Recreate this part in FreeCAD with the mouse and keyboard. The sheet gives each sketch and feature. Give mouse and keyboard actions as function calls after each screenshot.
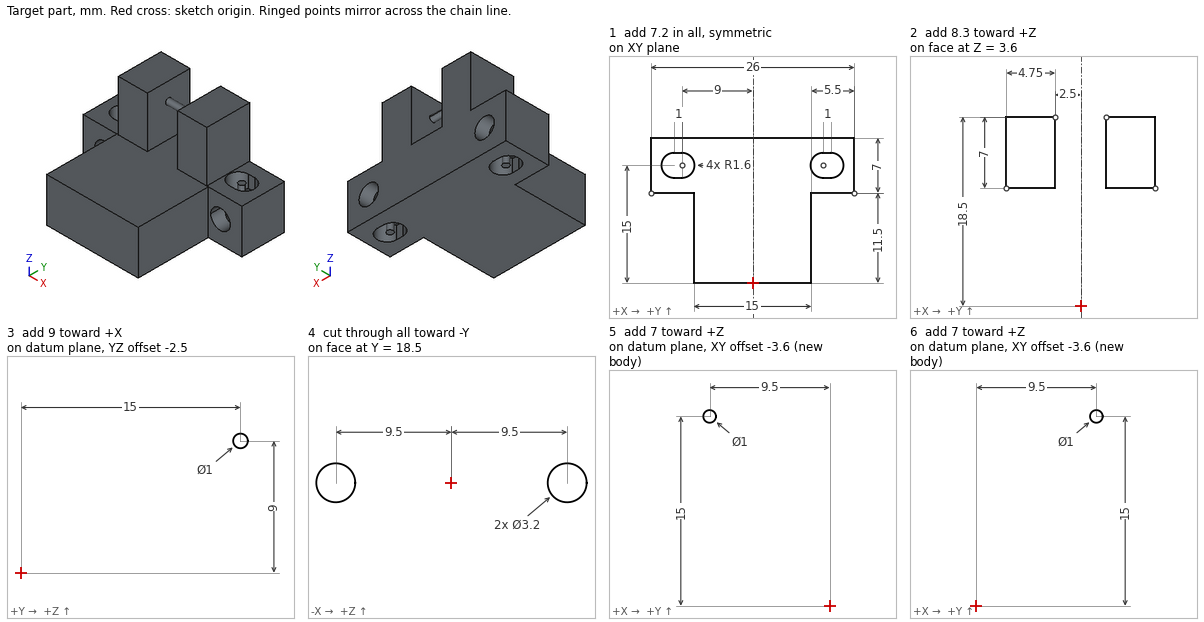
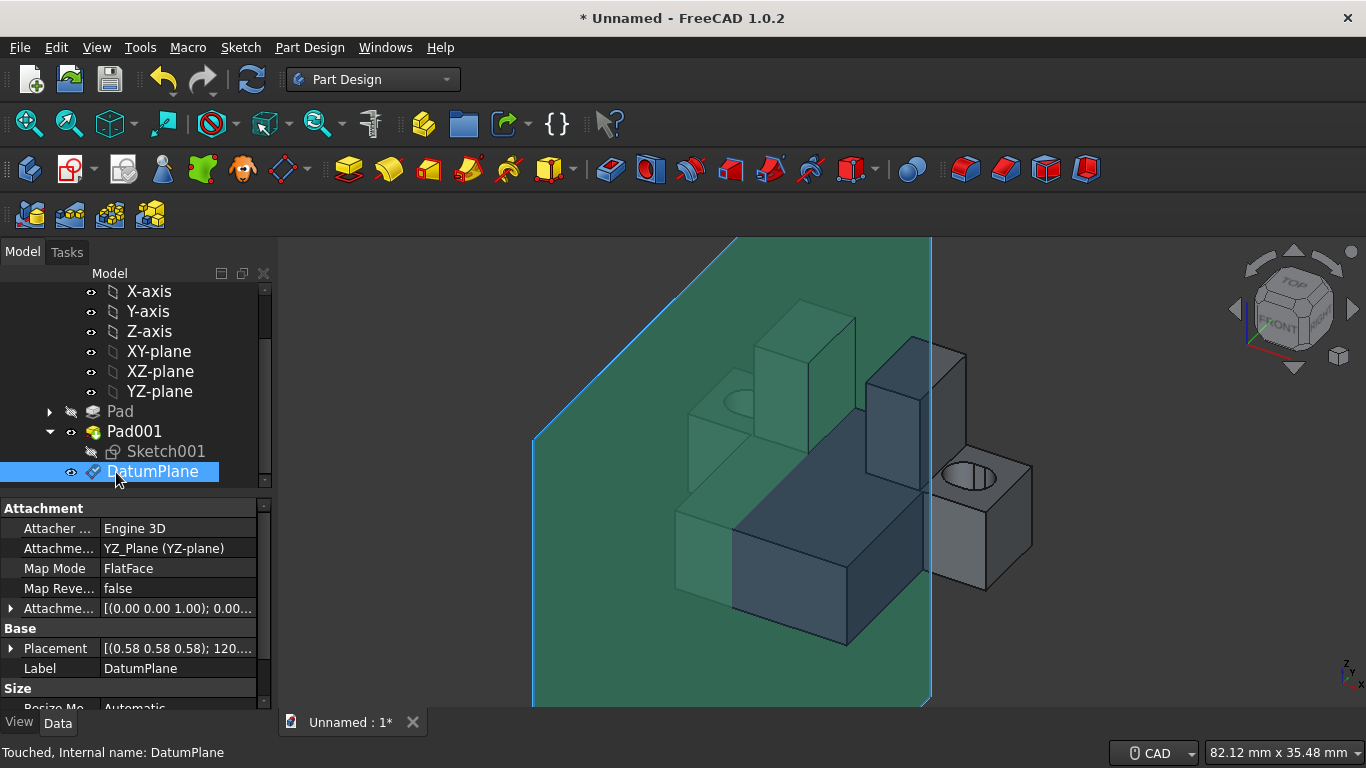
click(70, 170)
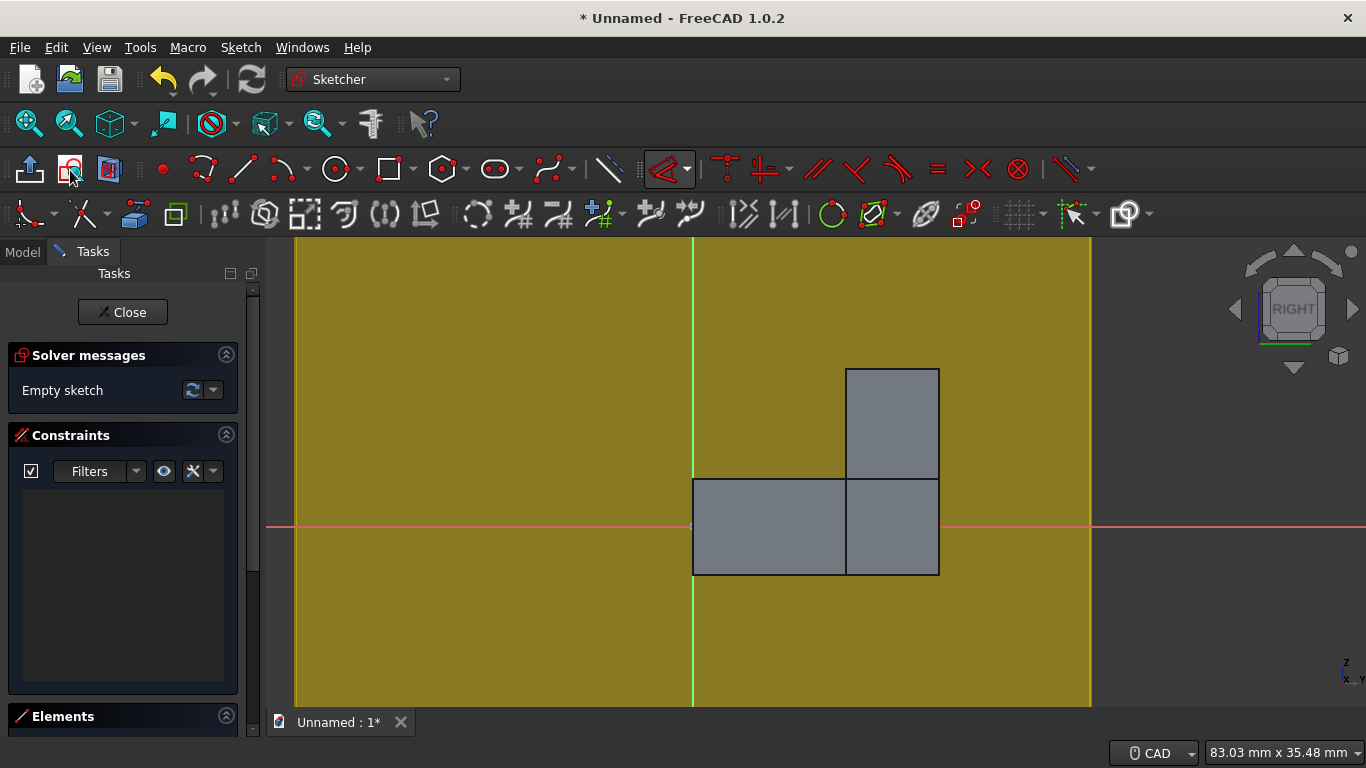
key(q)
key(s)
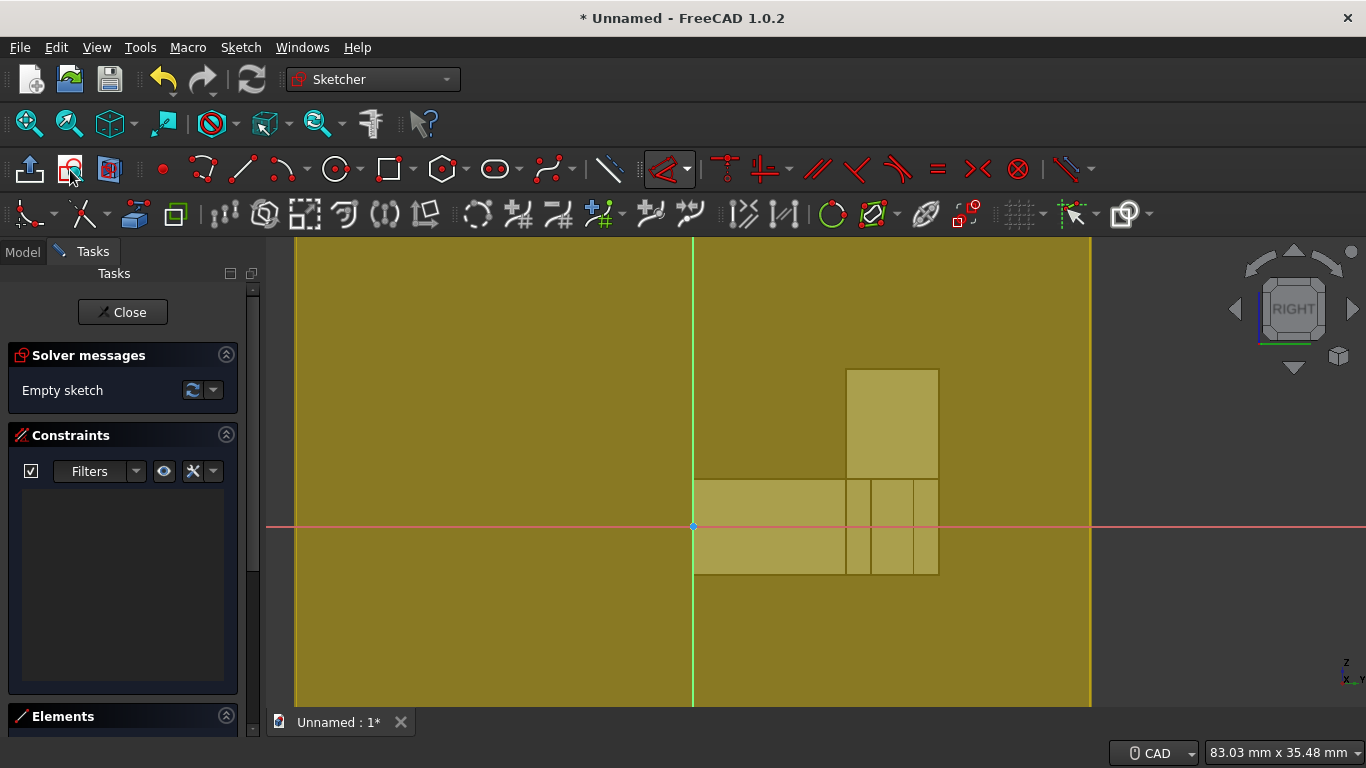
scroll(900, 404, up, 15)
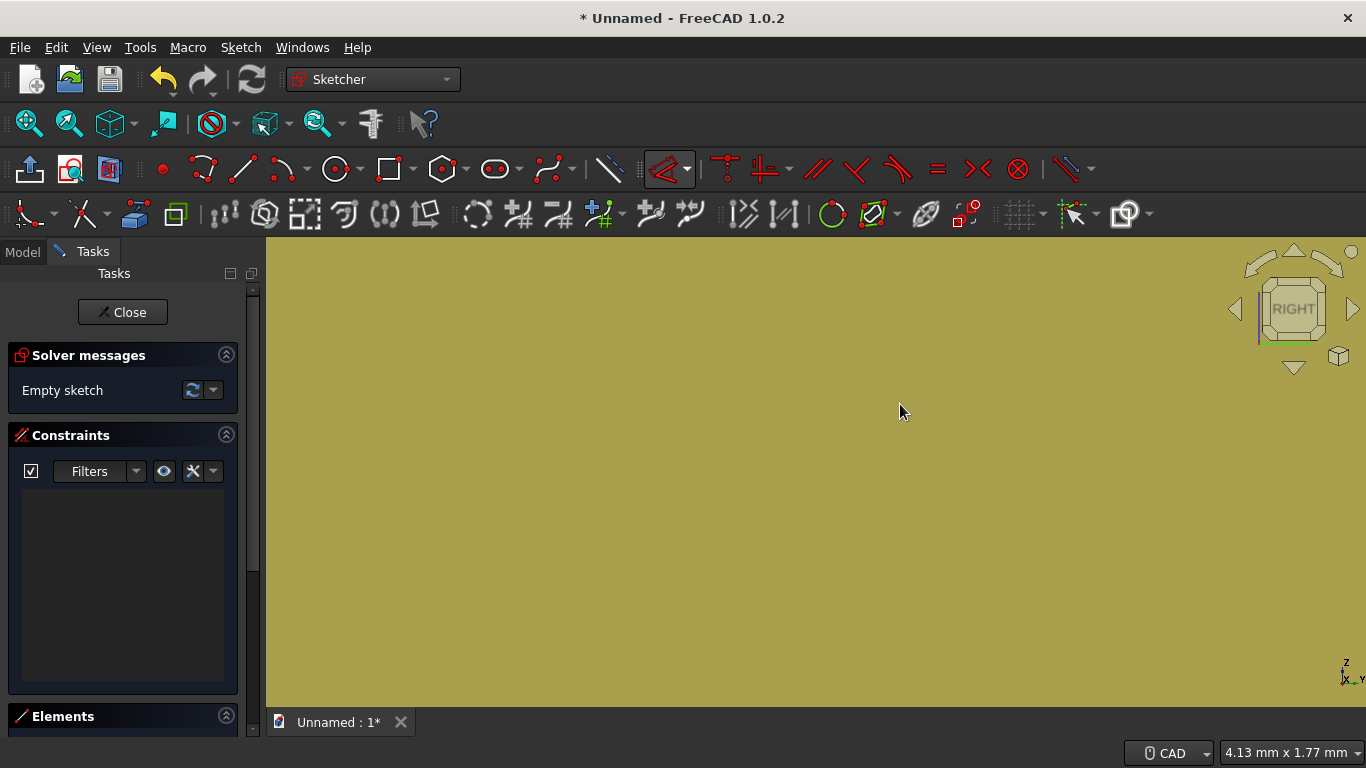
click(336, 170)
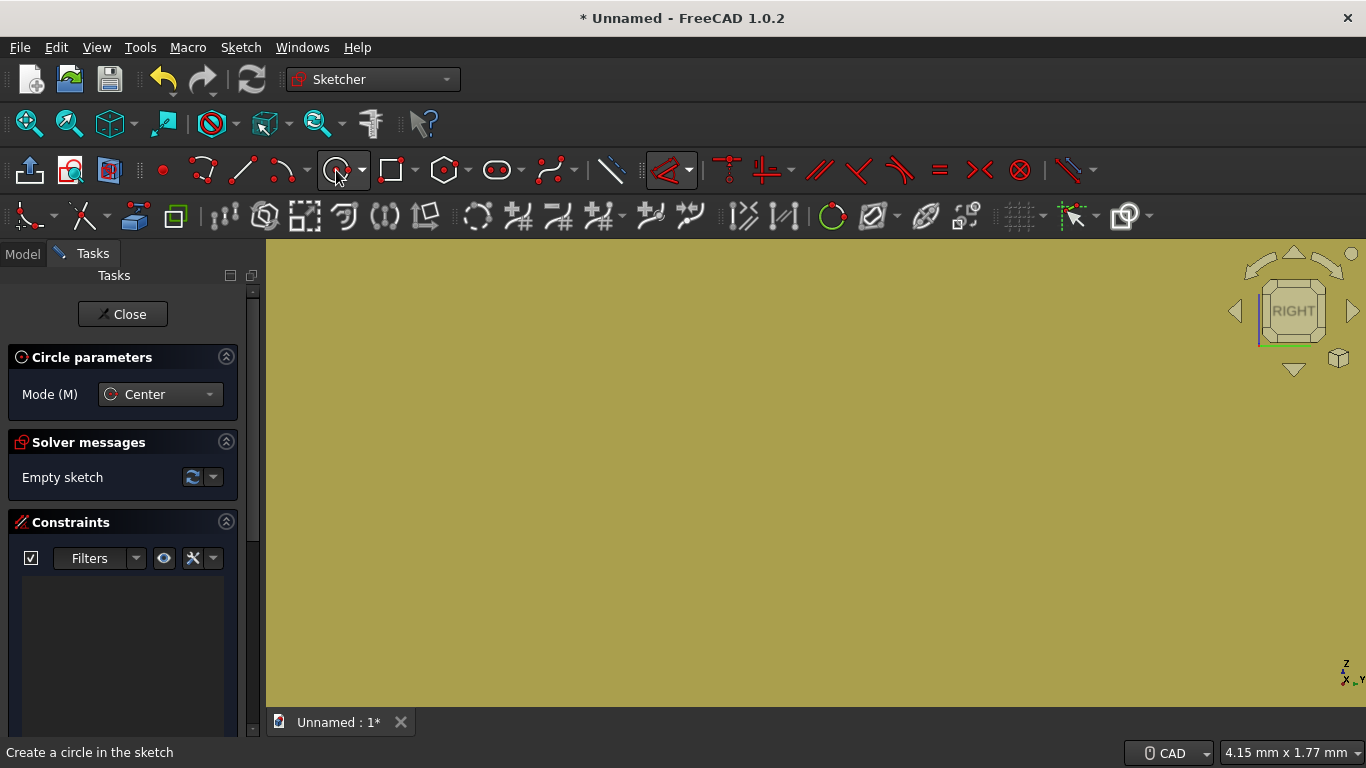
click(732, 473)
click(826, 380)
key(Escape)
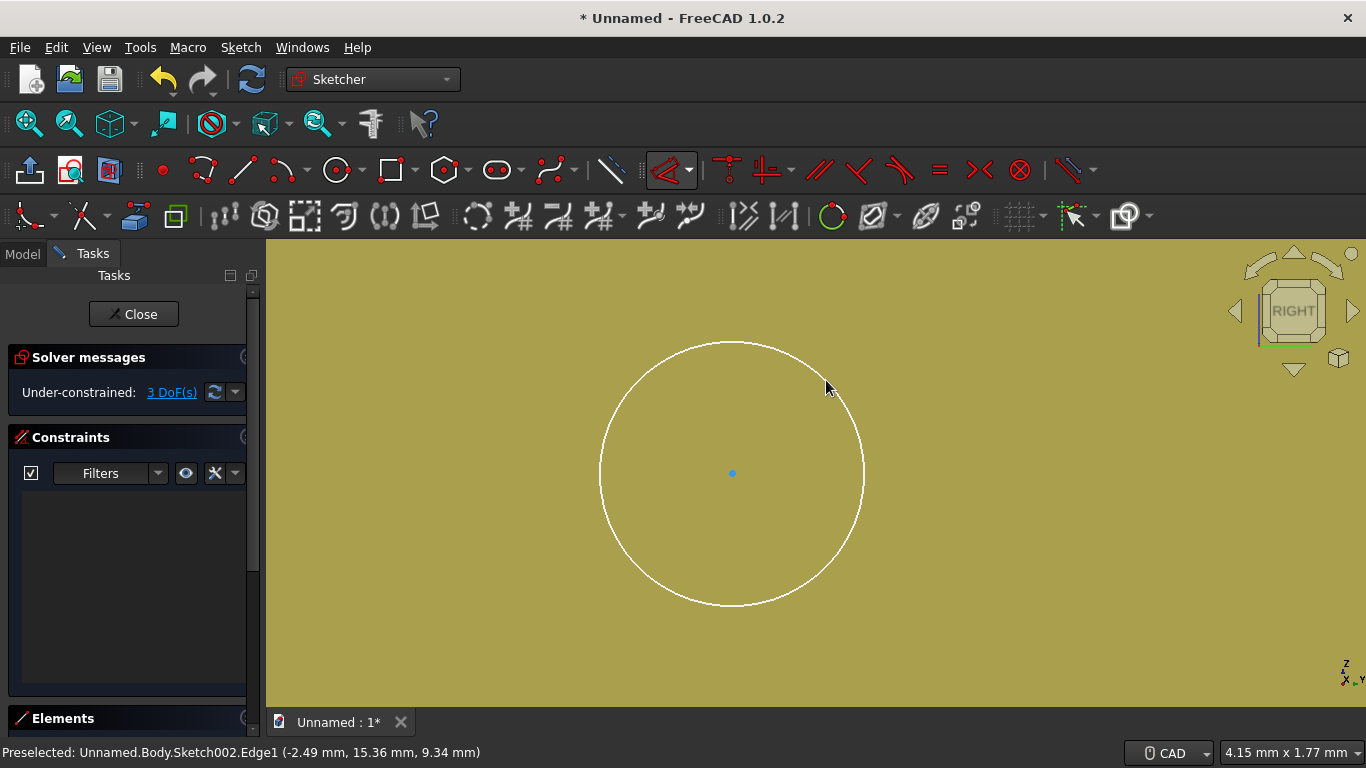
click(825, 380)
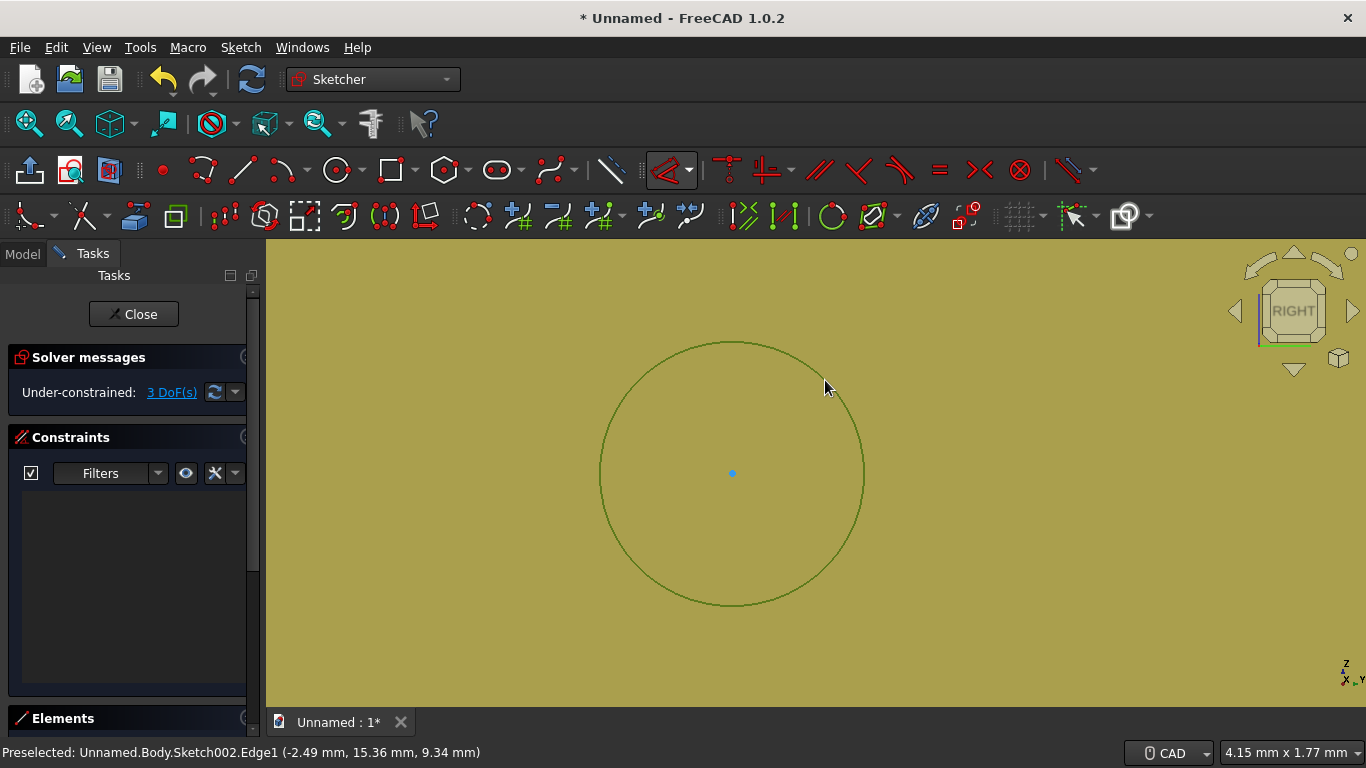
click(692, 170)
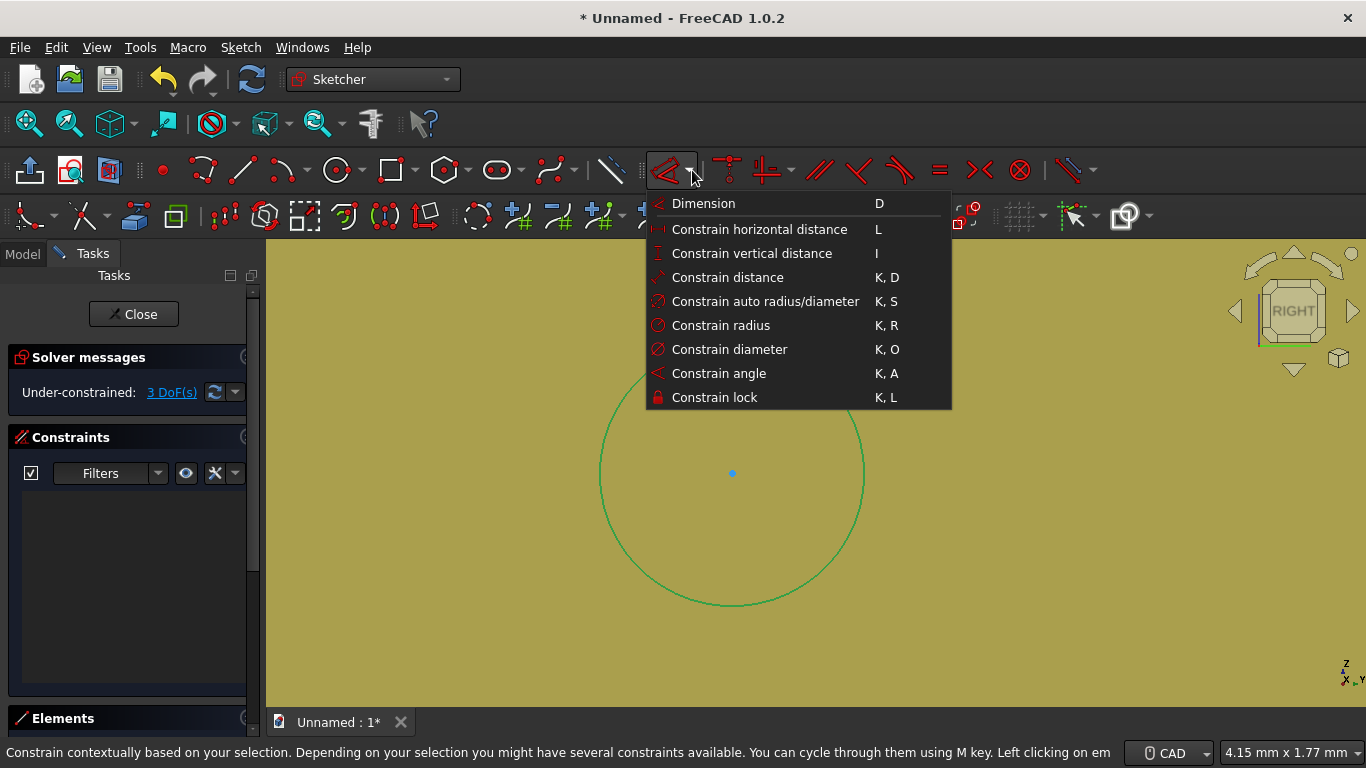
click(799, 349)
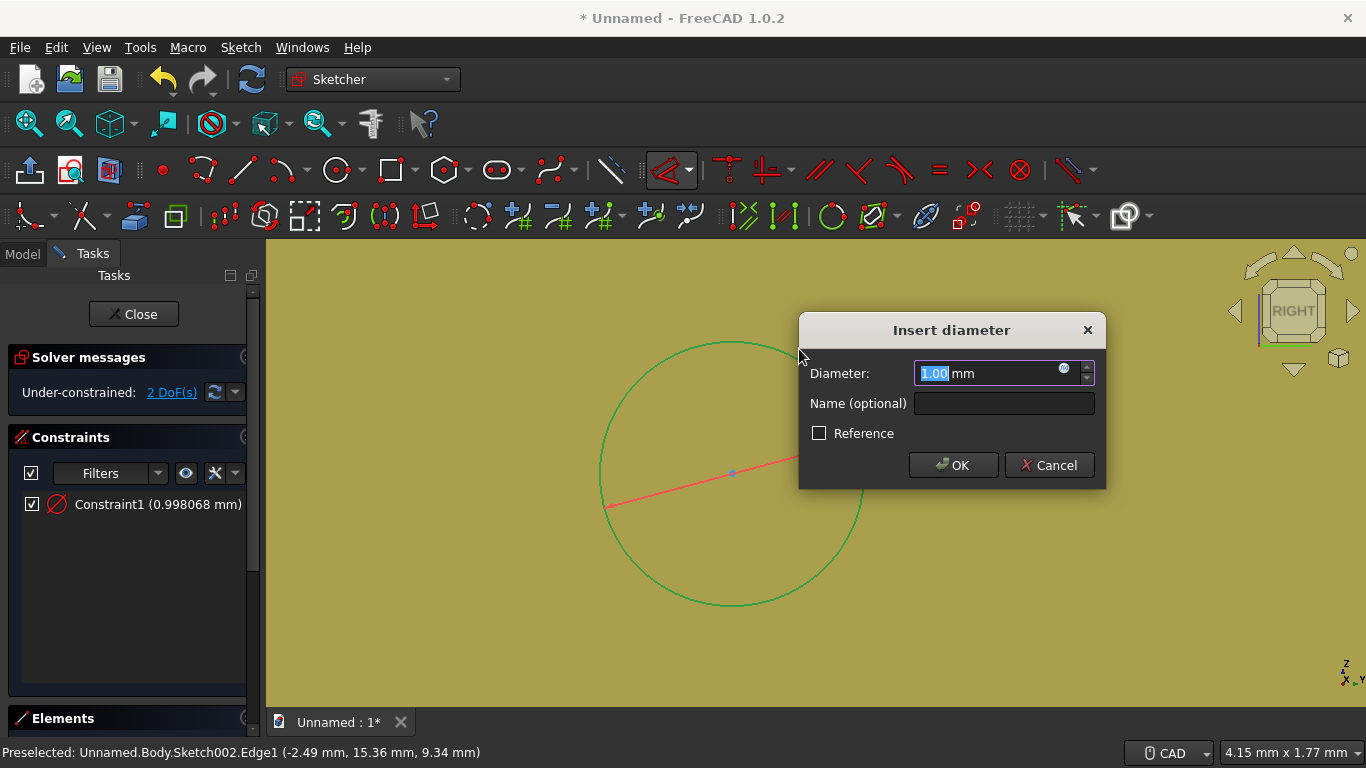
text(1)
key(Return)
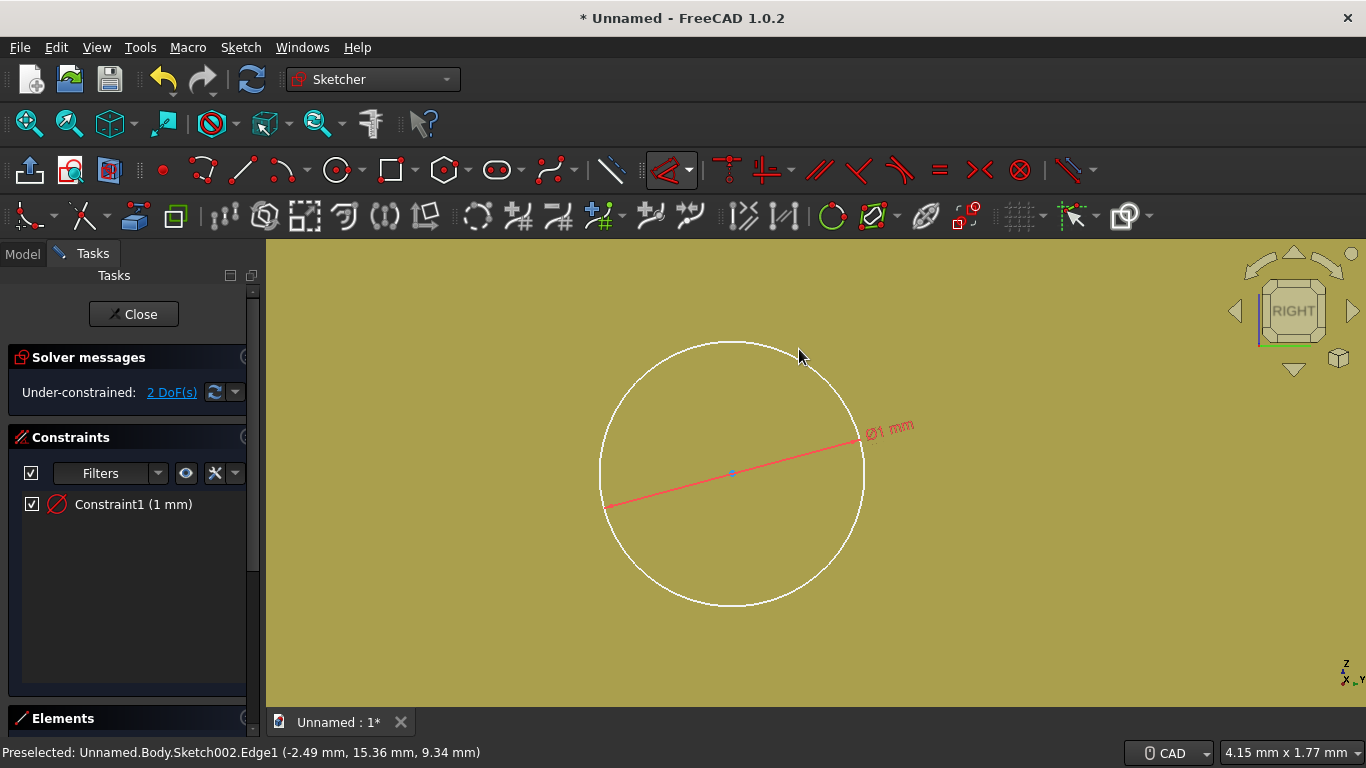
click(732, 474)